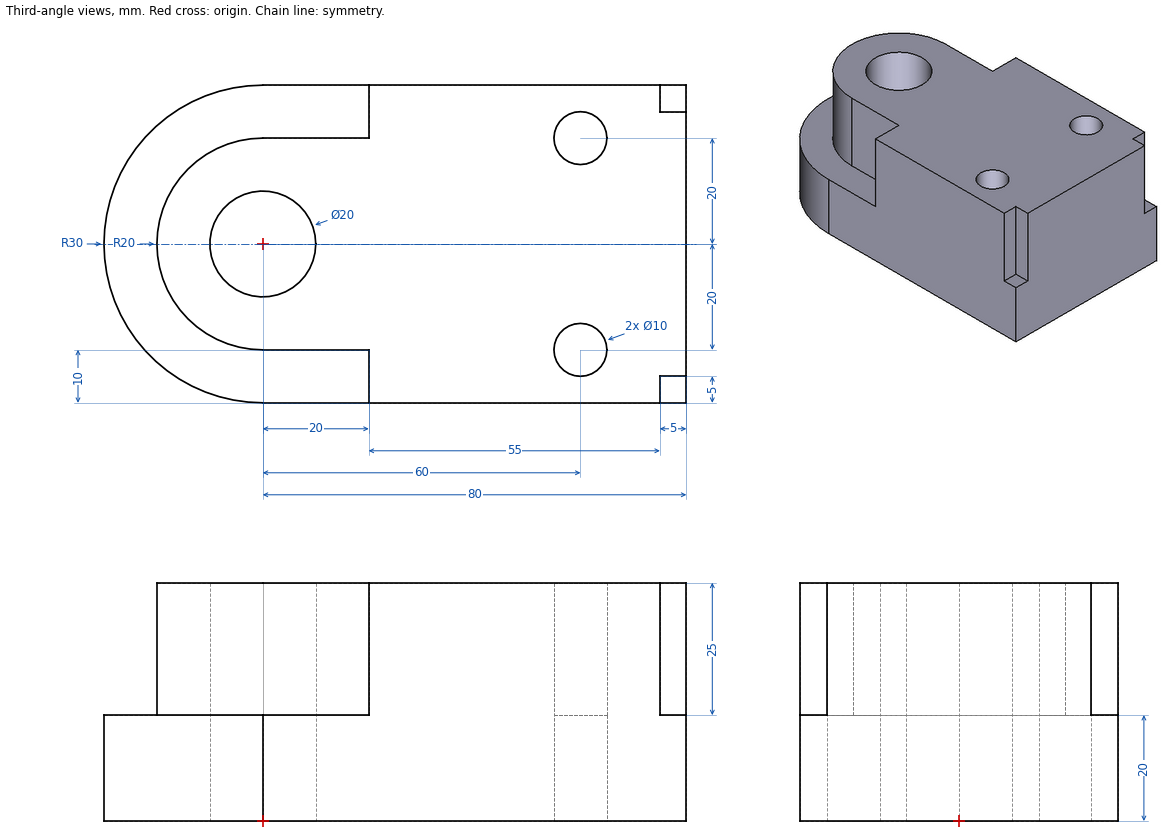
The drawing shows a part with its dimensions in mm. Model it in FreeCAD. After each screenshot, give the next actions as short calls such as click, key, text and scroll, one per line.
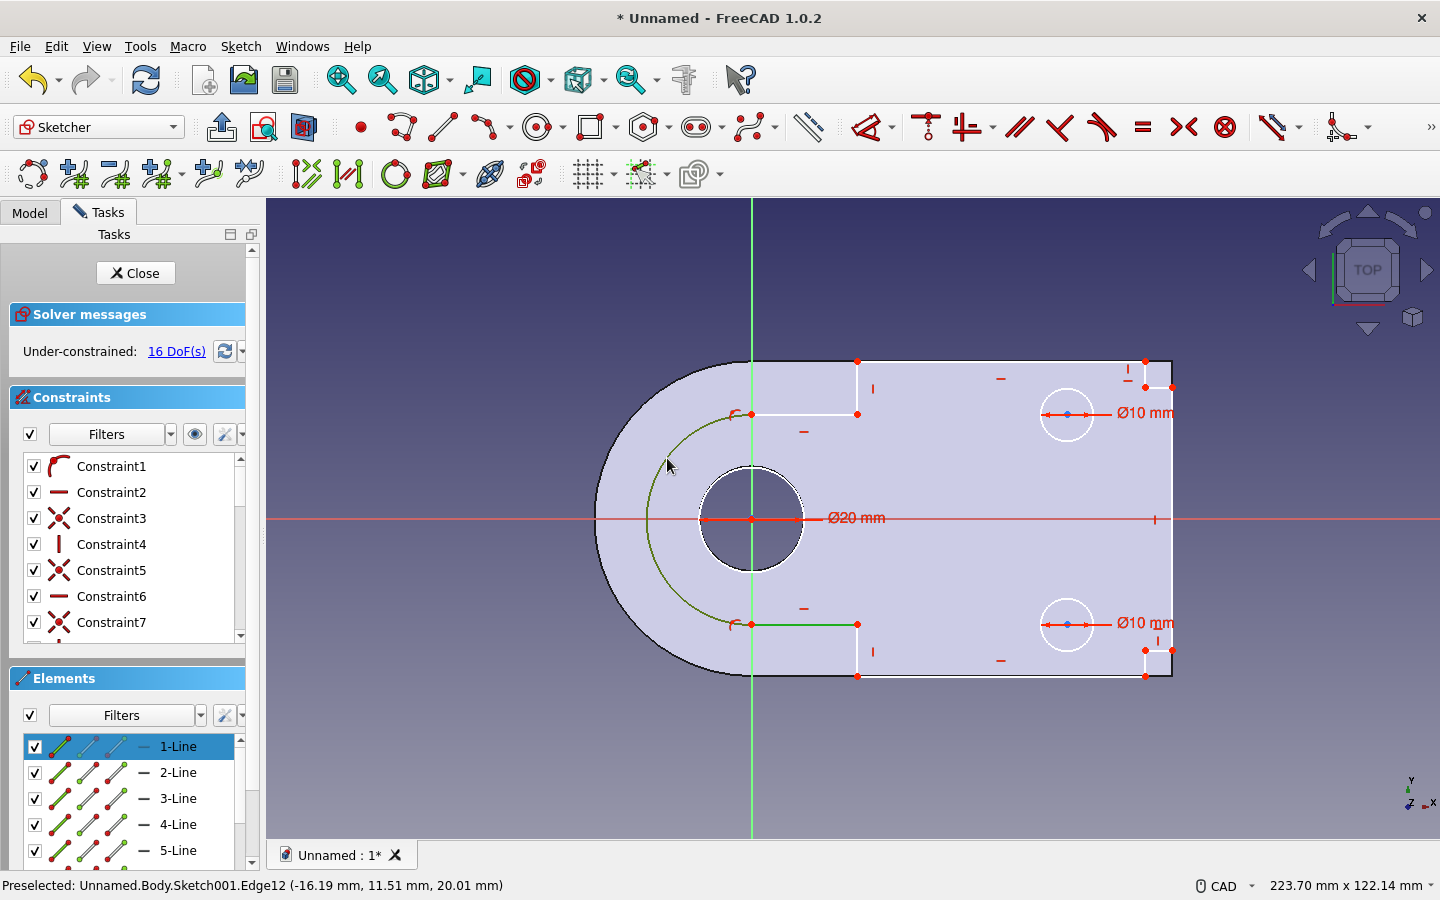
key(t)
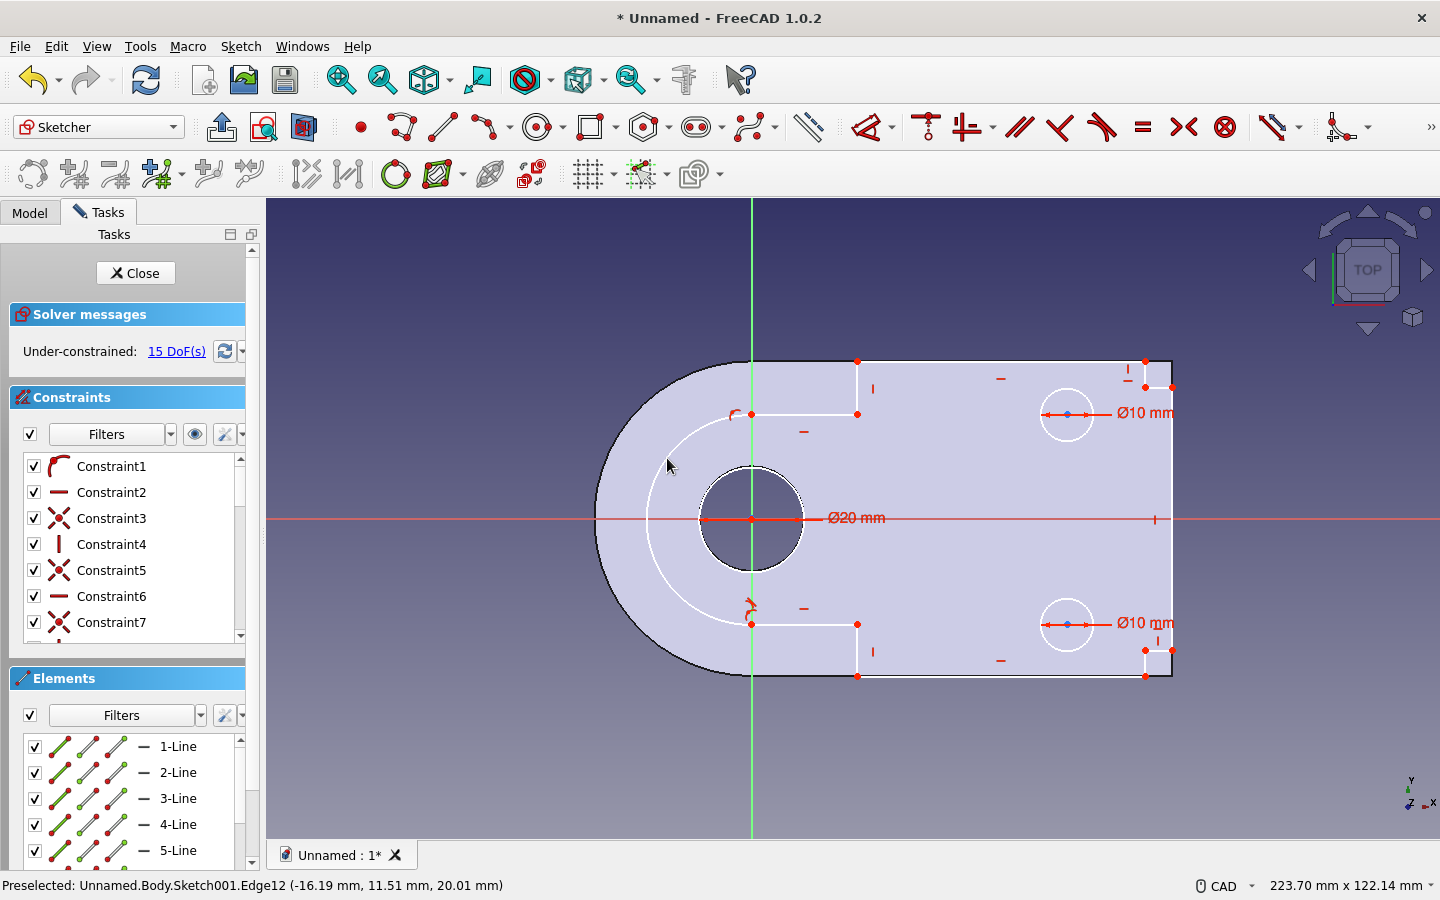
click(752, 520)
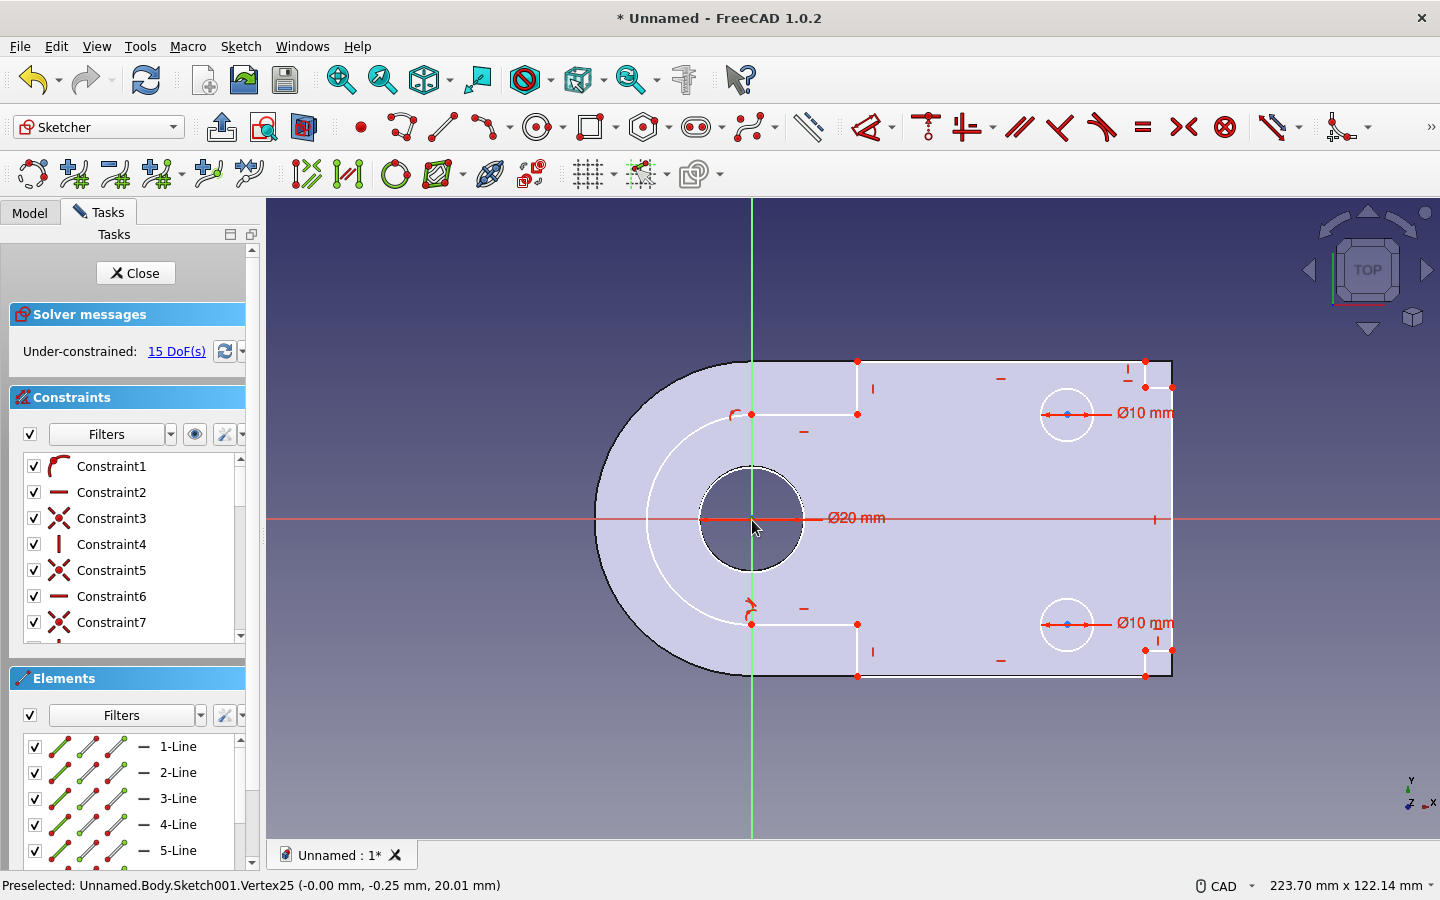
click(364, 519)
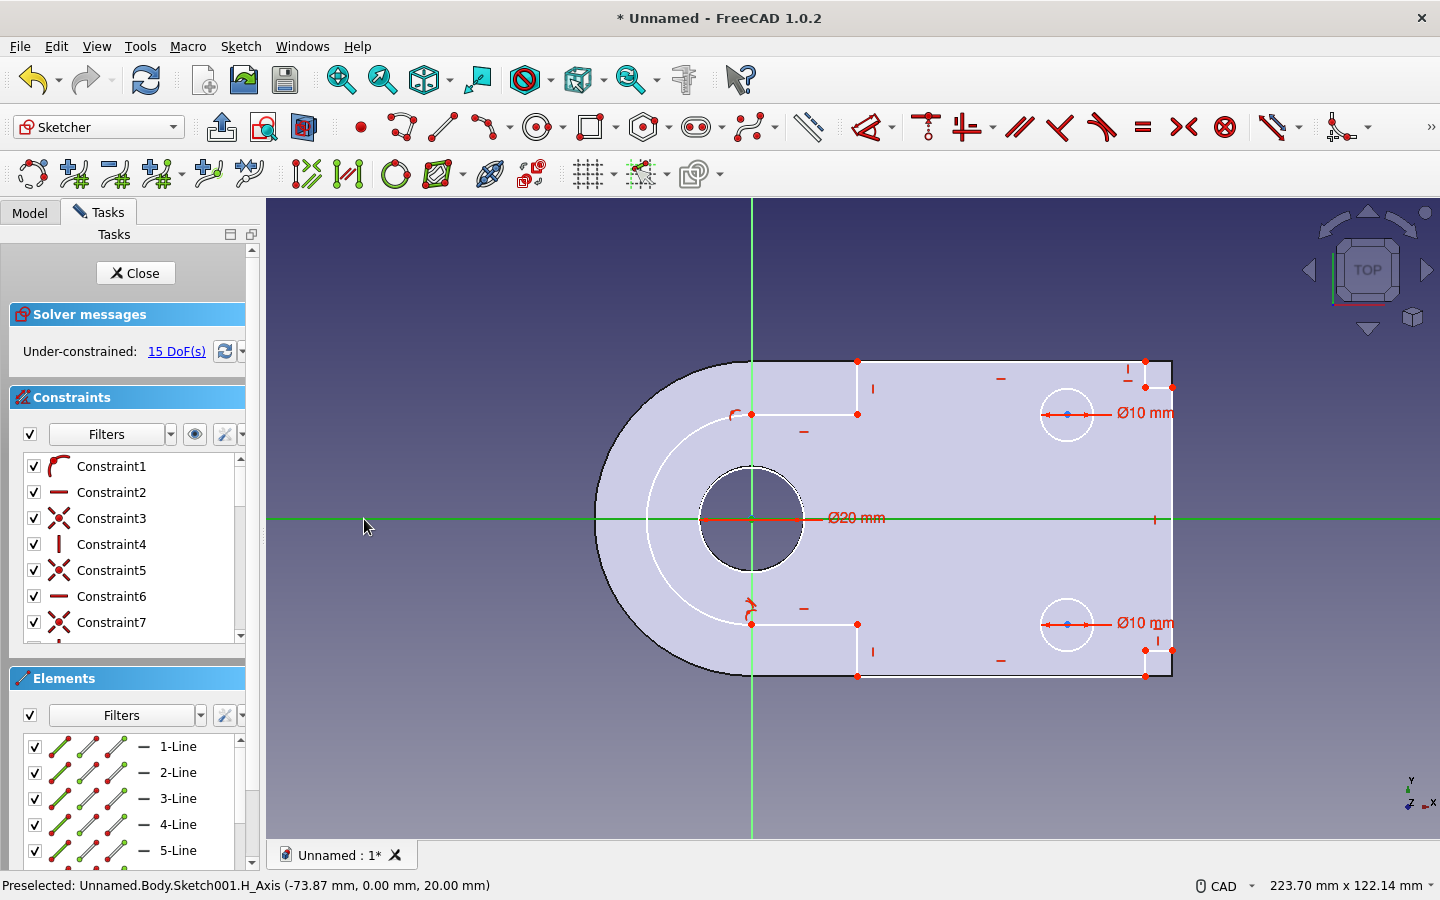
click(926, 128)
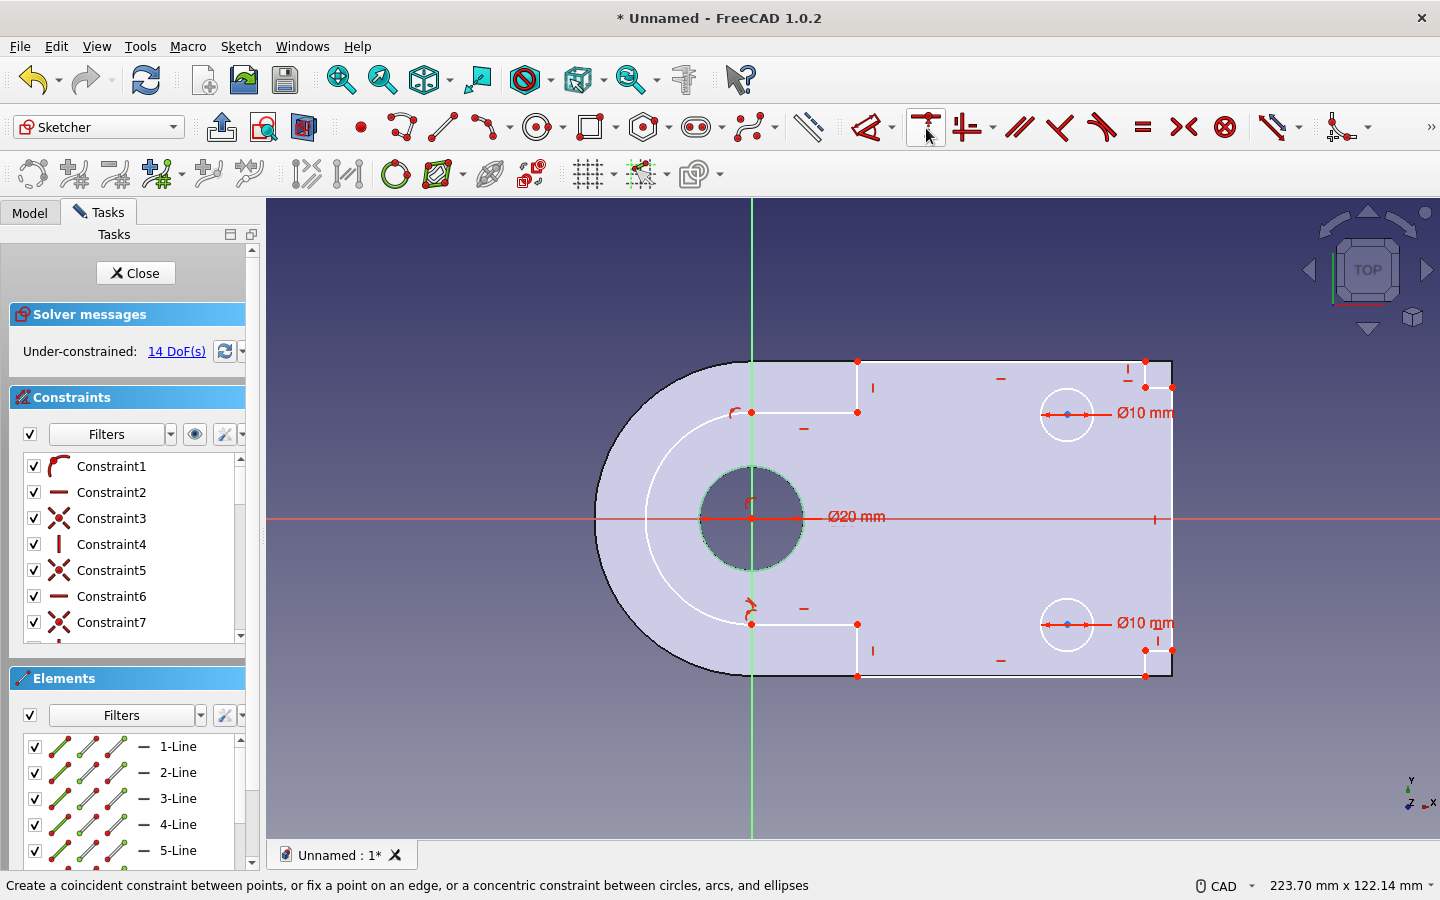
click(1067, 625)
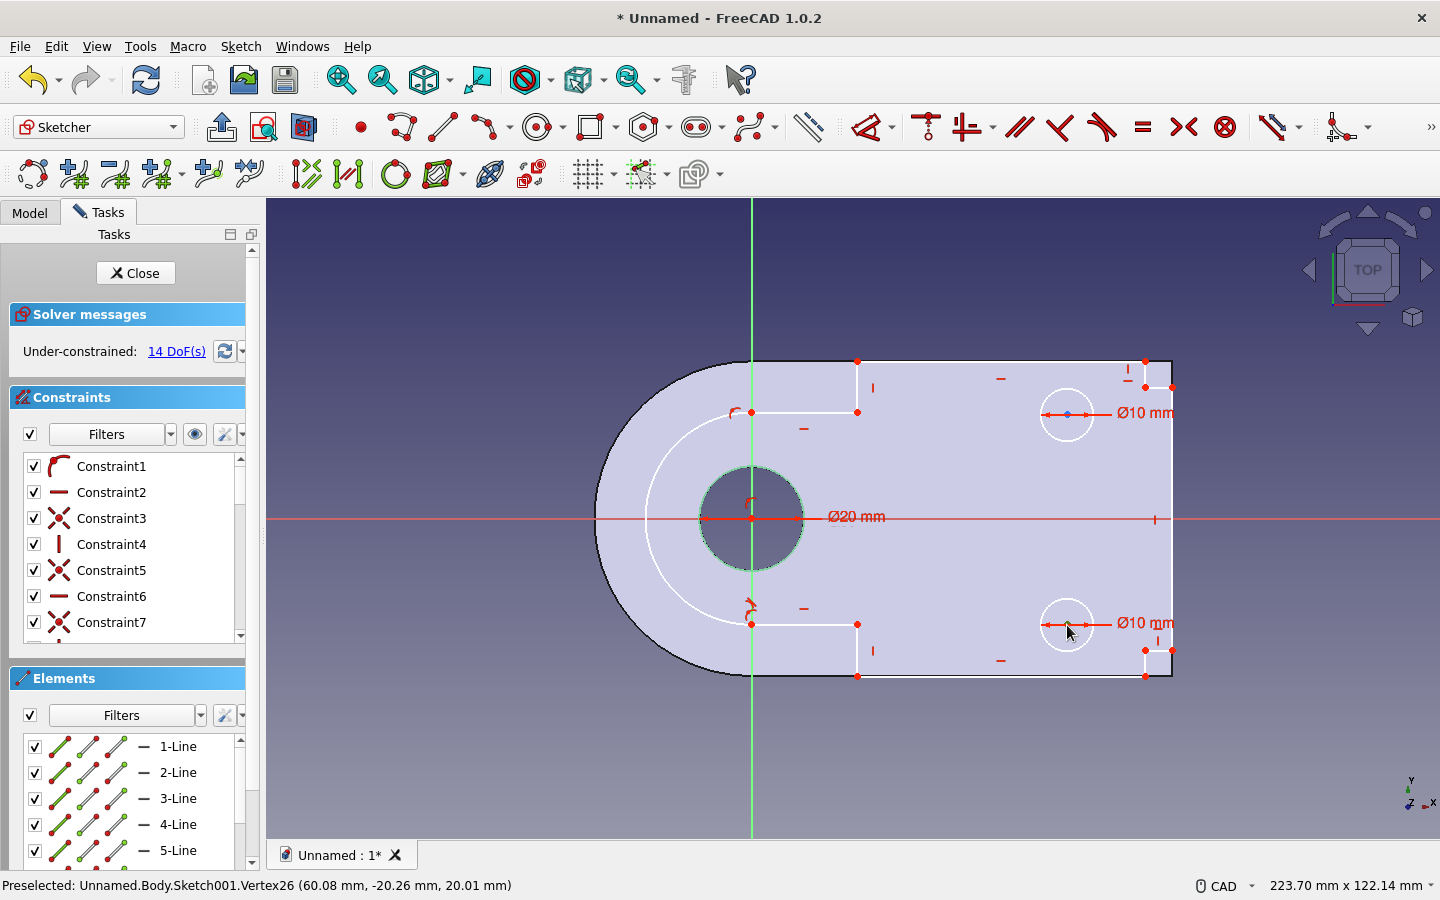
click(1067, 415)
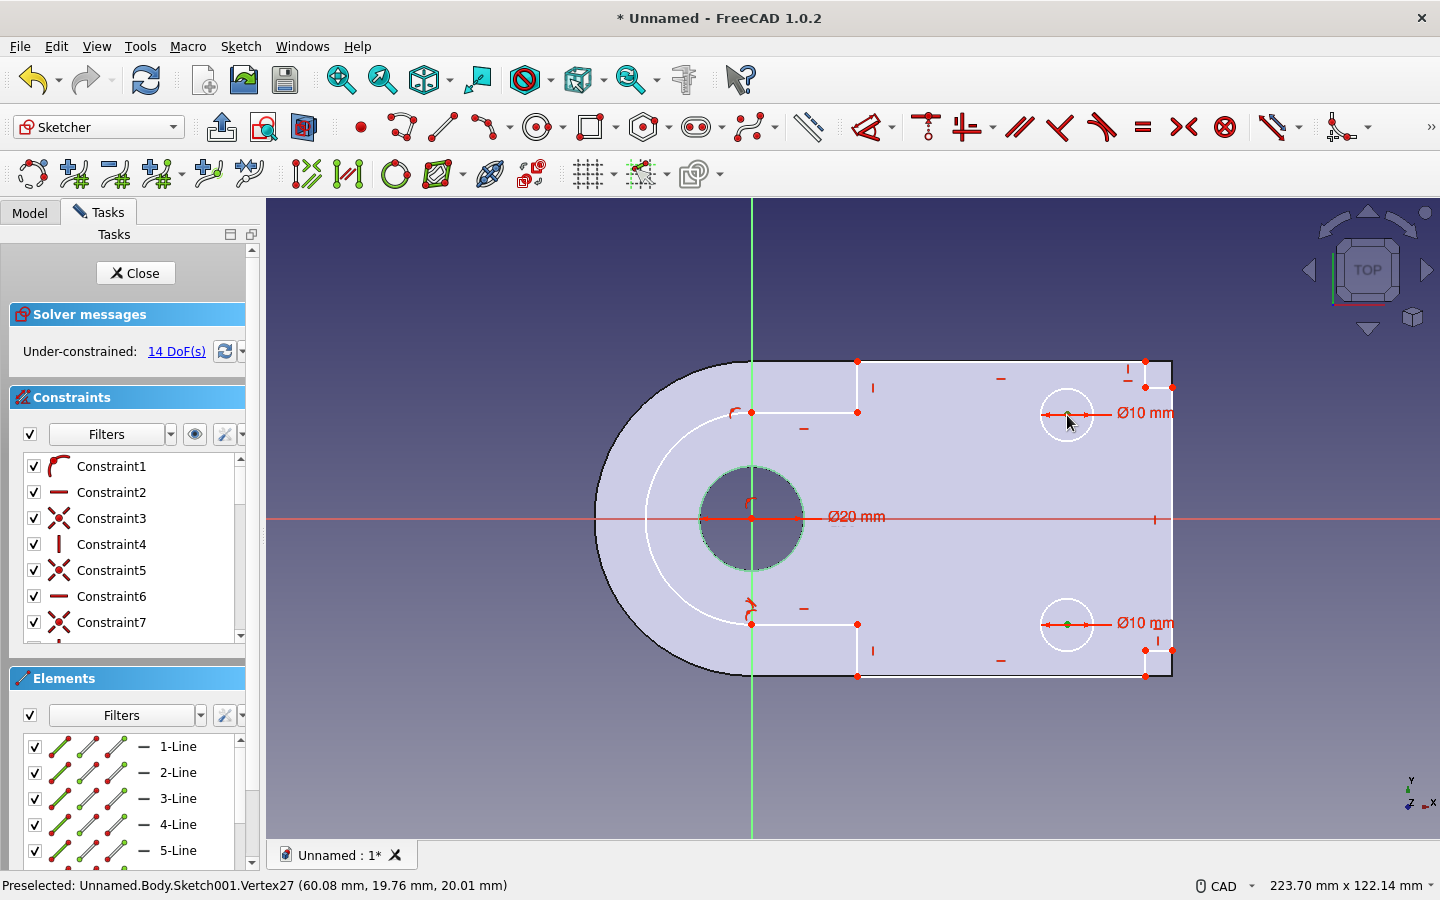
click(364, 519)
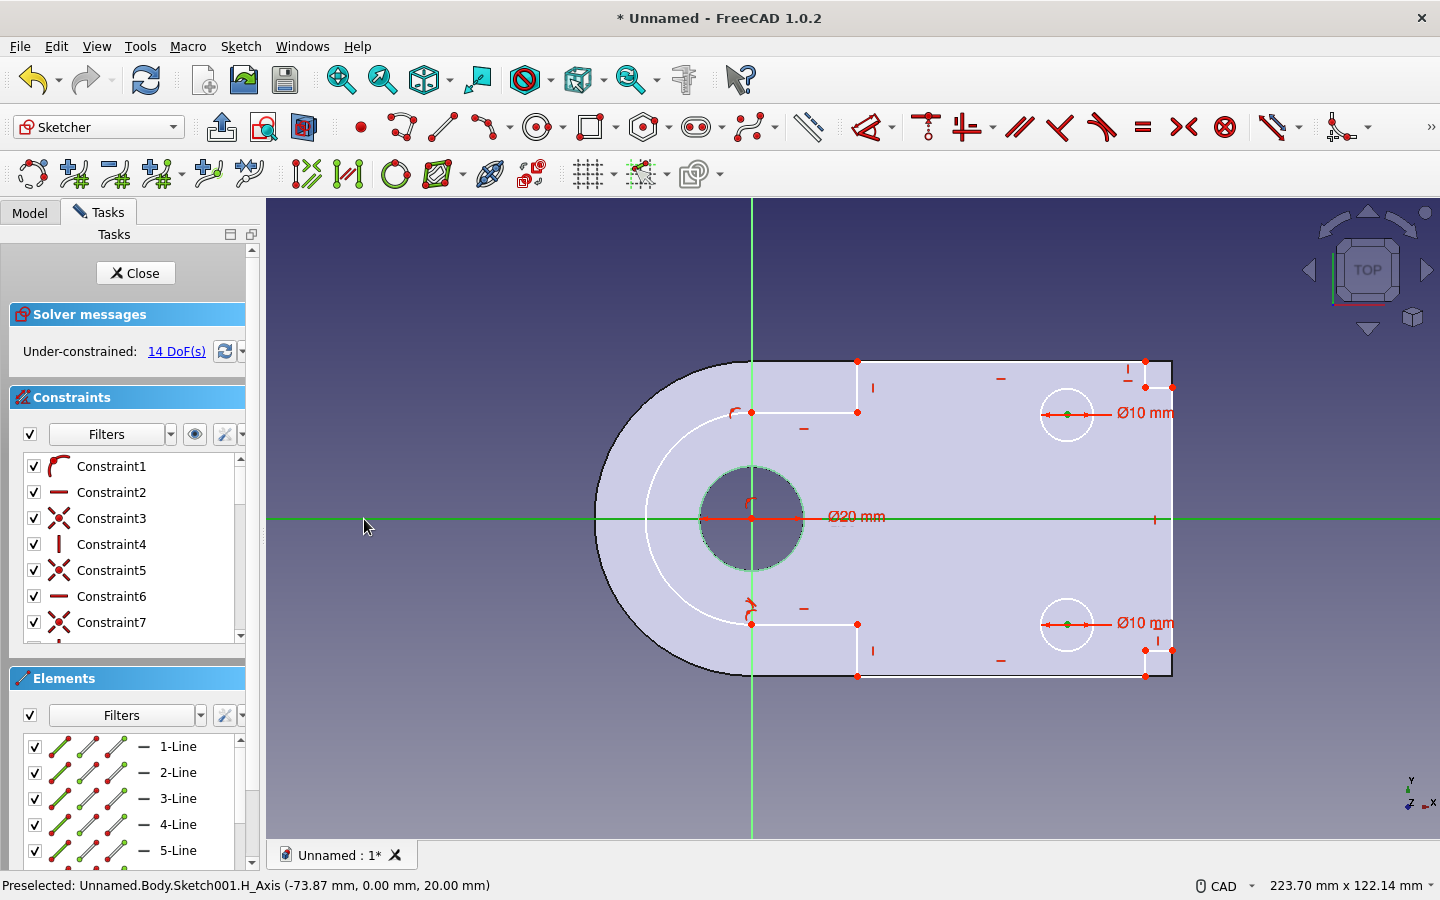
click(1184, 128)